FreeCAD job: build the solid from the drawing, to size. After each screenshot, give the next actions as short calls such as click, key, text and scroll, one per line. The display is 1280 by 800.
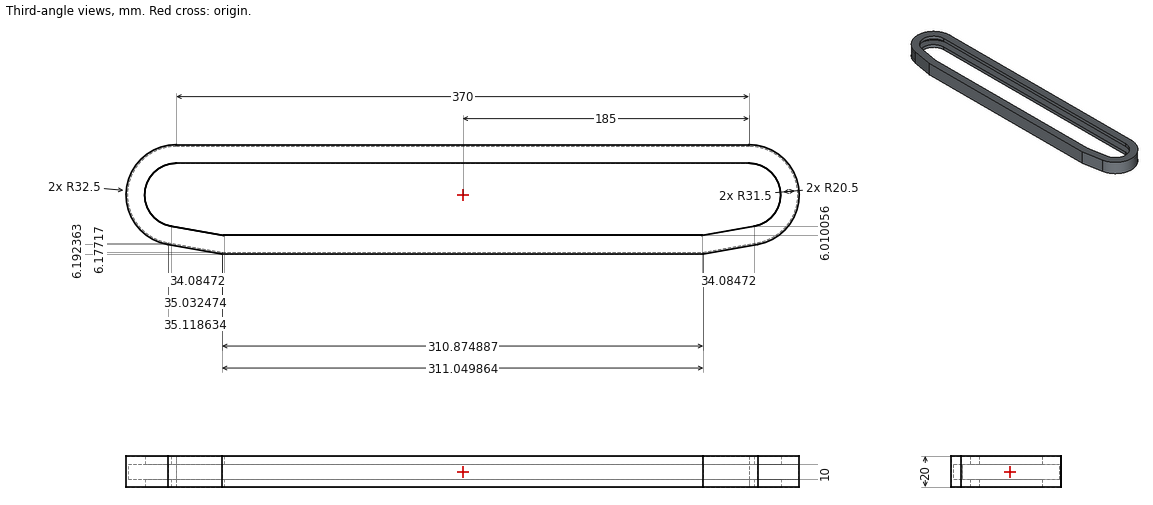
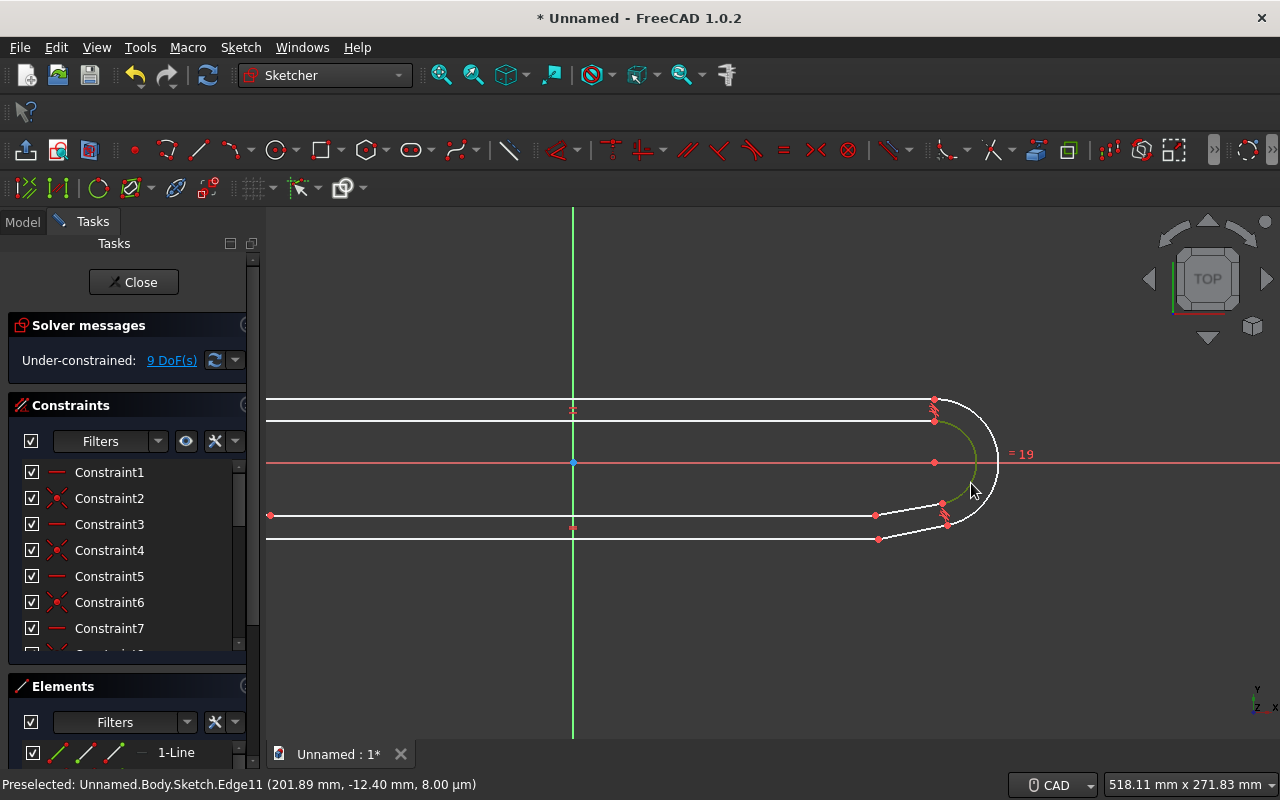
key(k)
key(r)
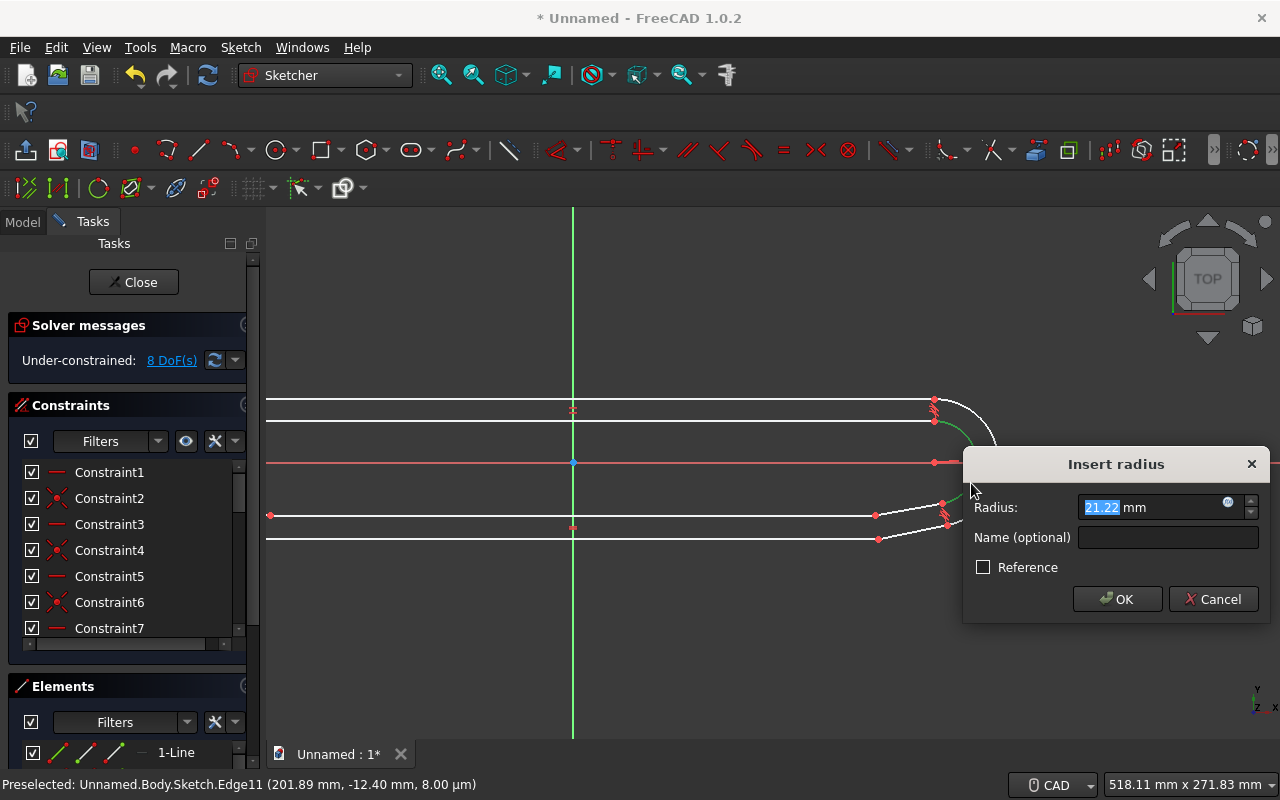
text(20.5)
key(Return)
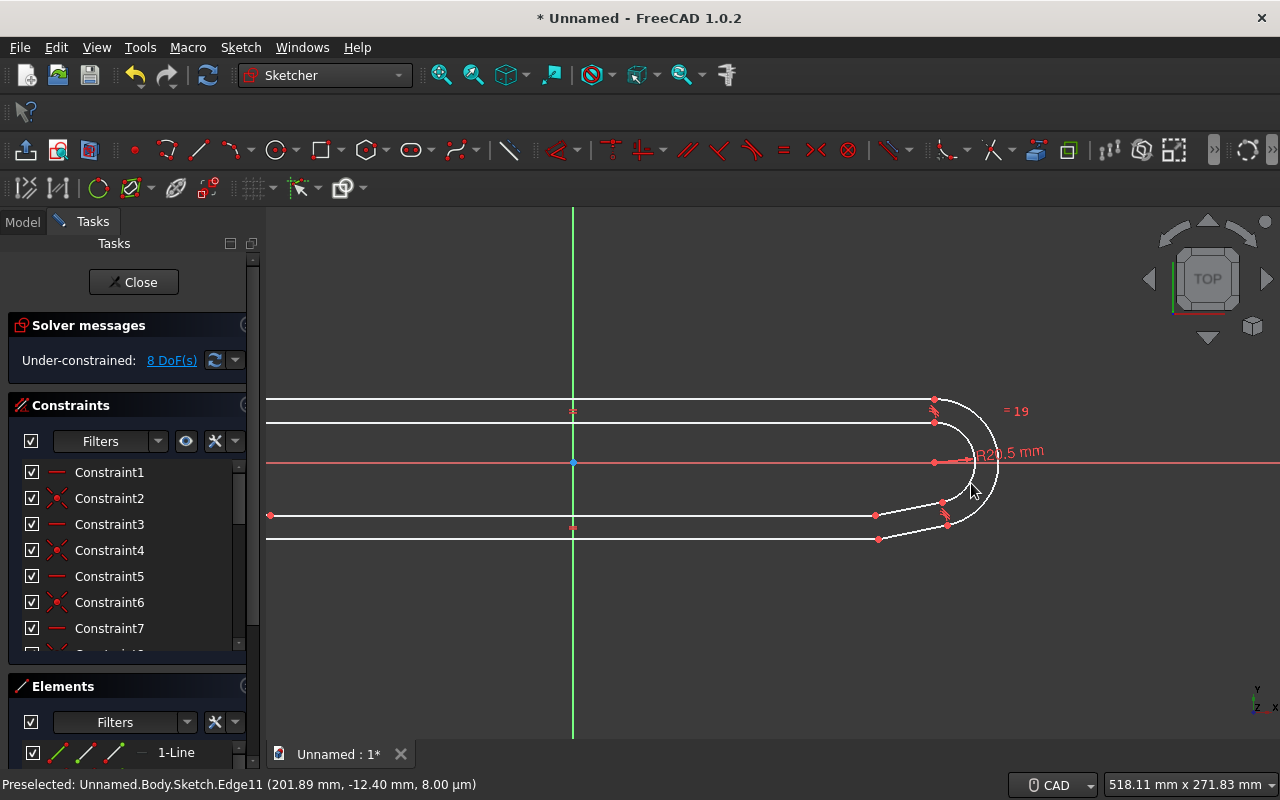
click(718, 399)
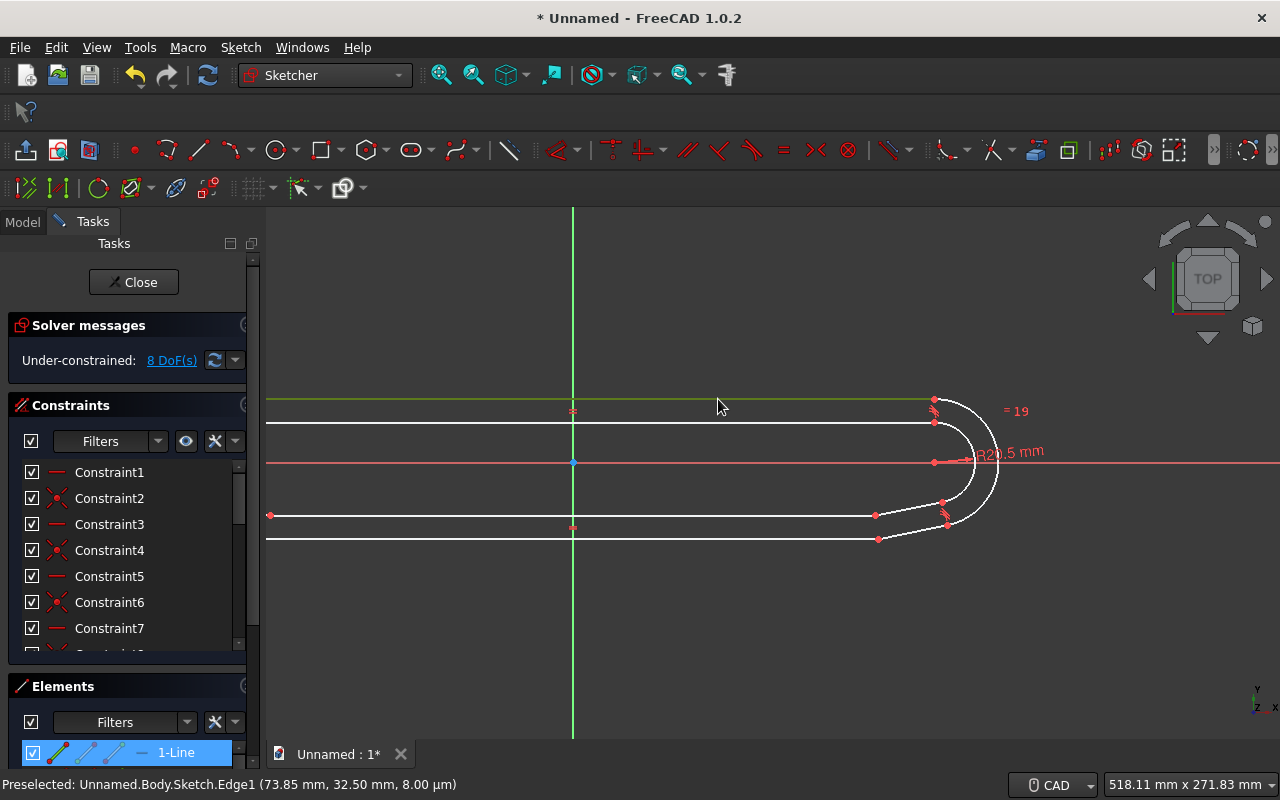
key(l)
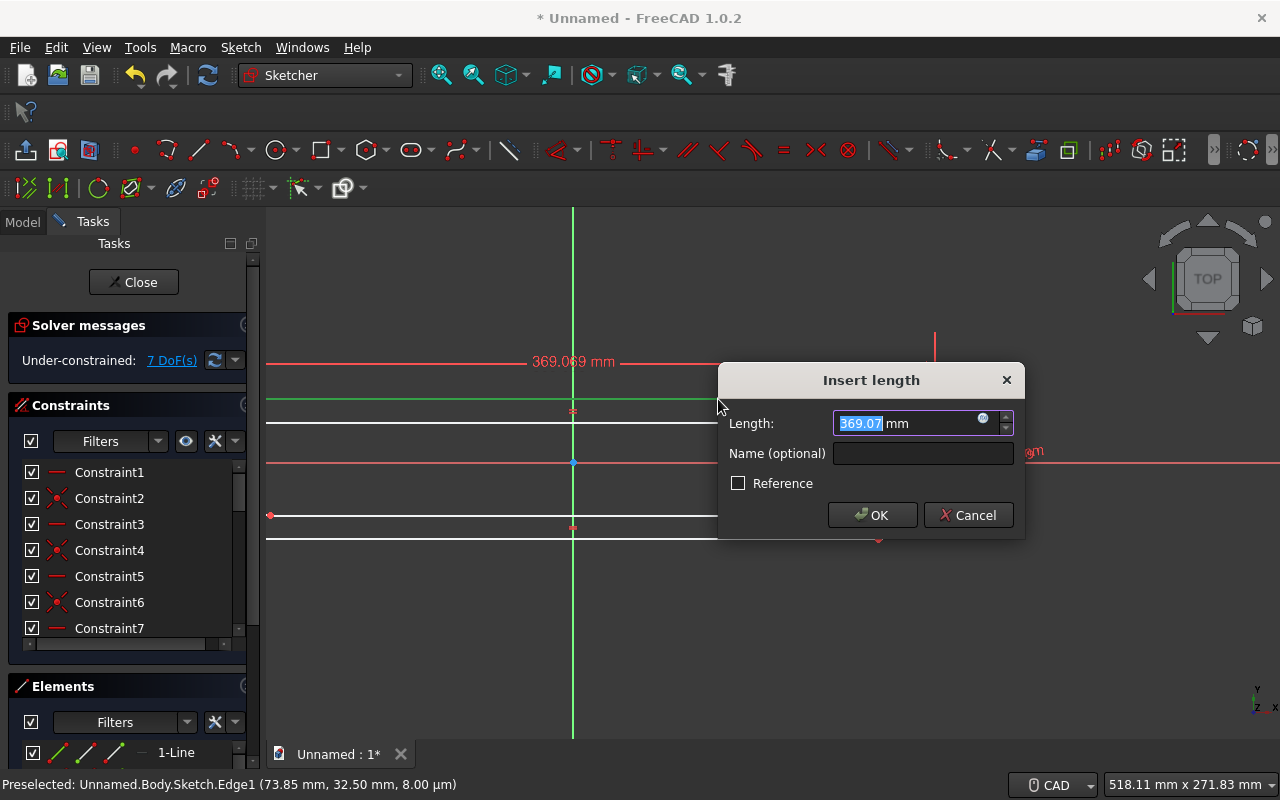
text(370)
key(Return)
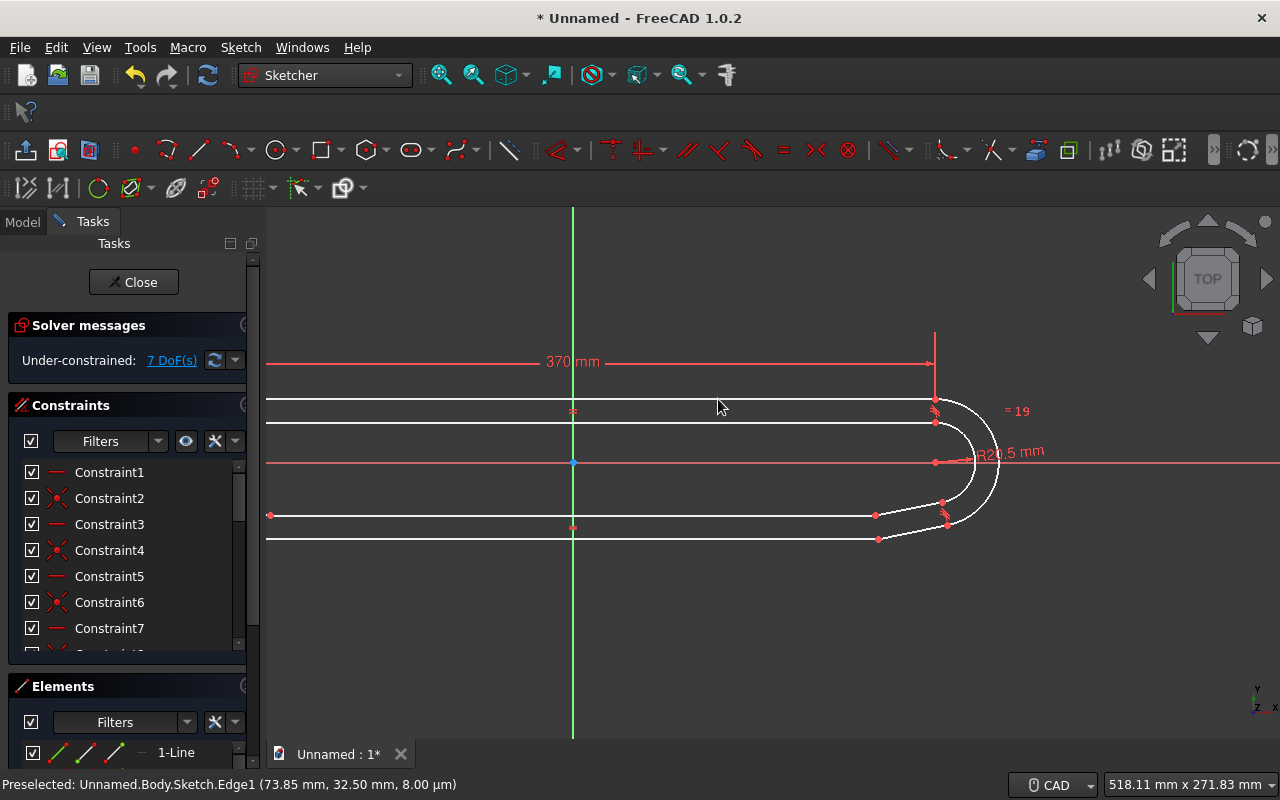
click(935, 399)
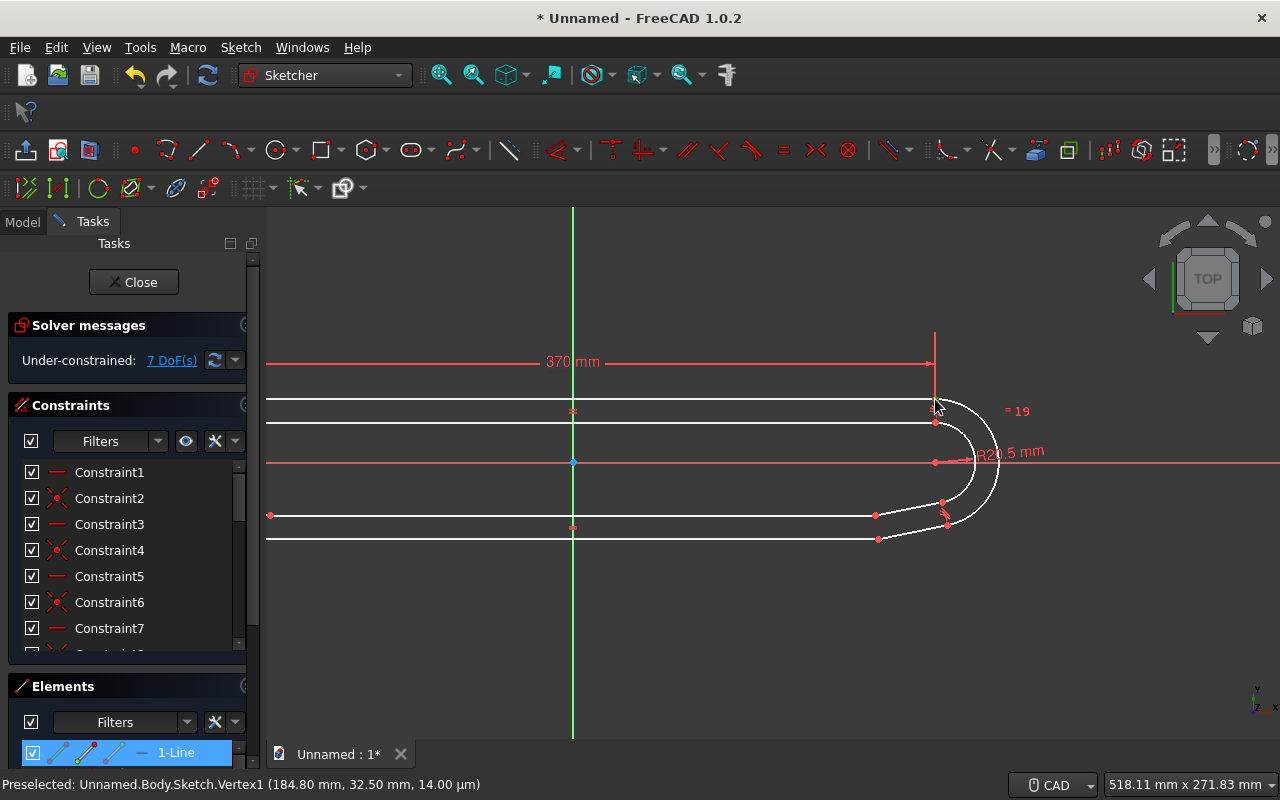
key(l)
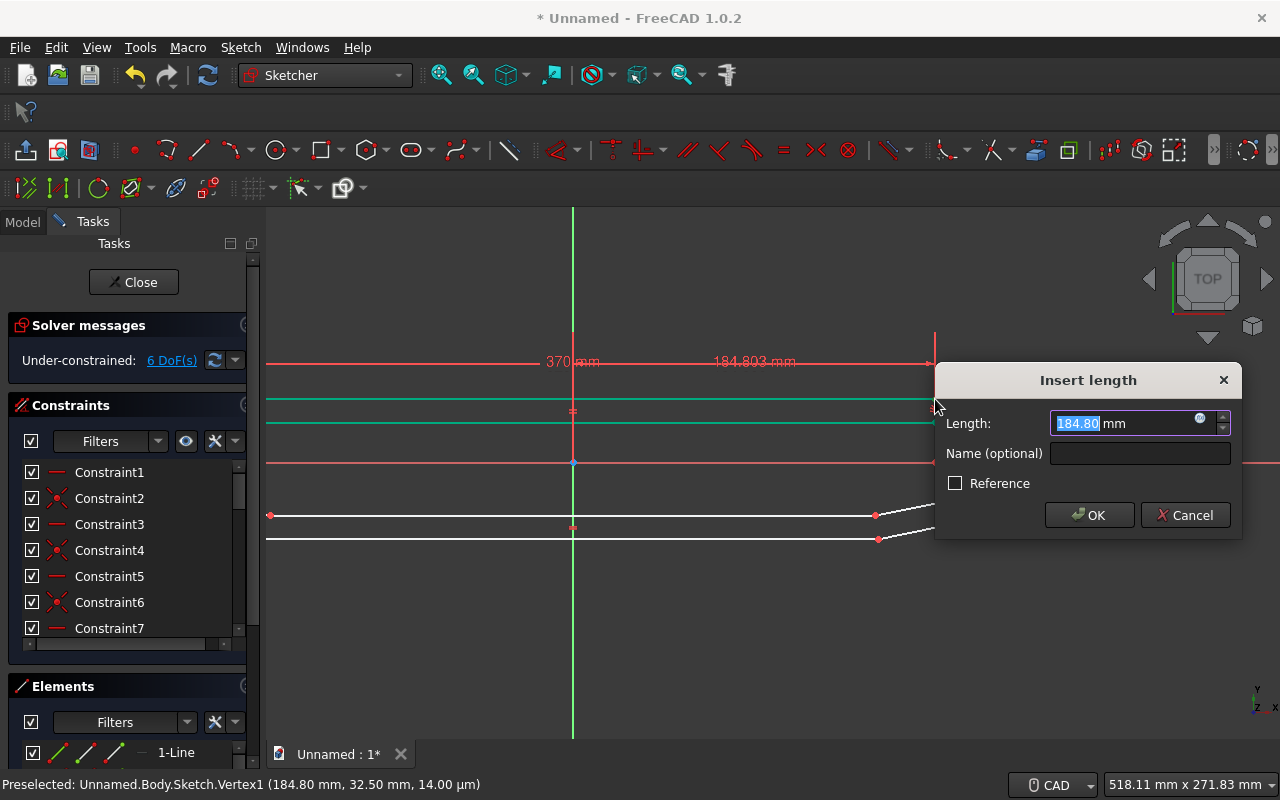
text(185)
key(Return)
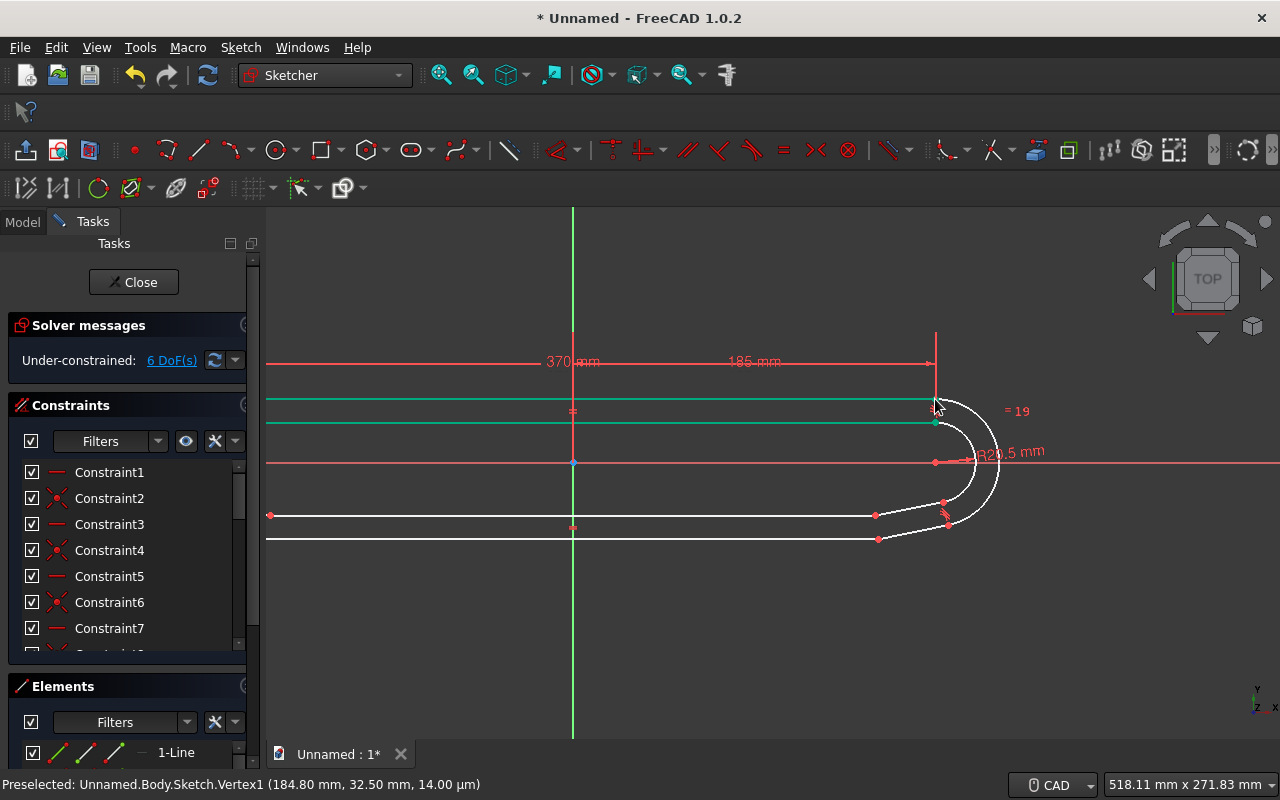
scroll(971, 482, down, 2)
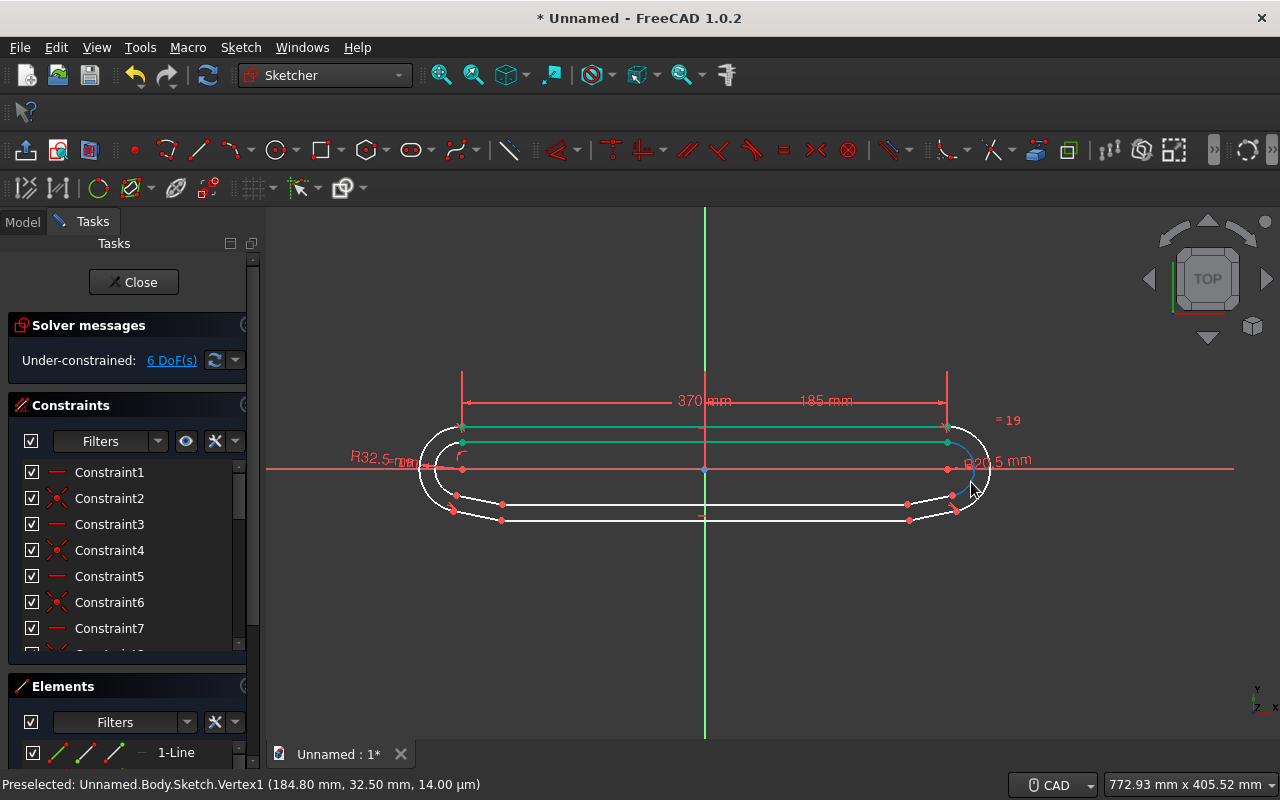
scroll(468, 514, up, 8)